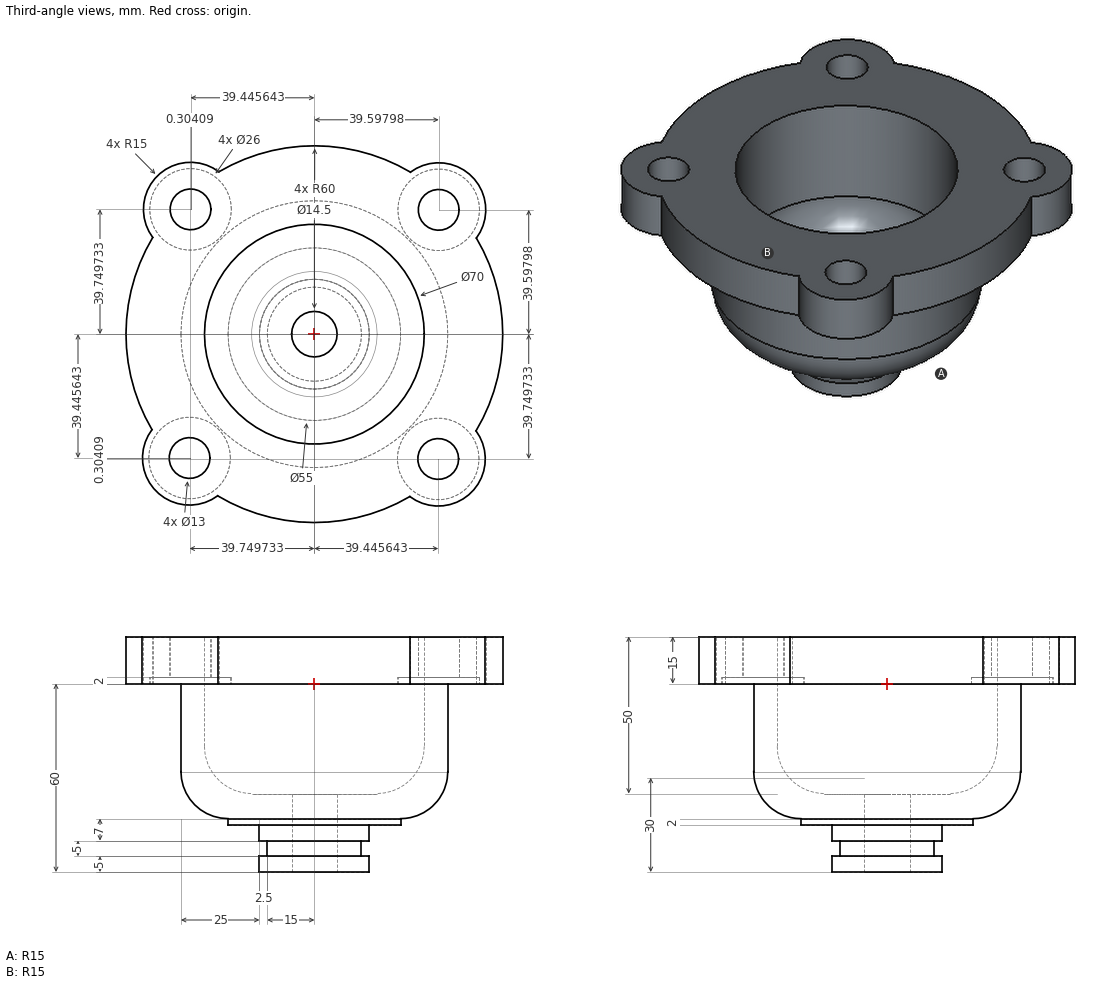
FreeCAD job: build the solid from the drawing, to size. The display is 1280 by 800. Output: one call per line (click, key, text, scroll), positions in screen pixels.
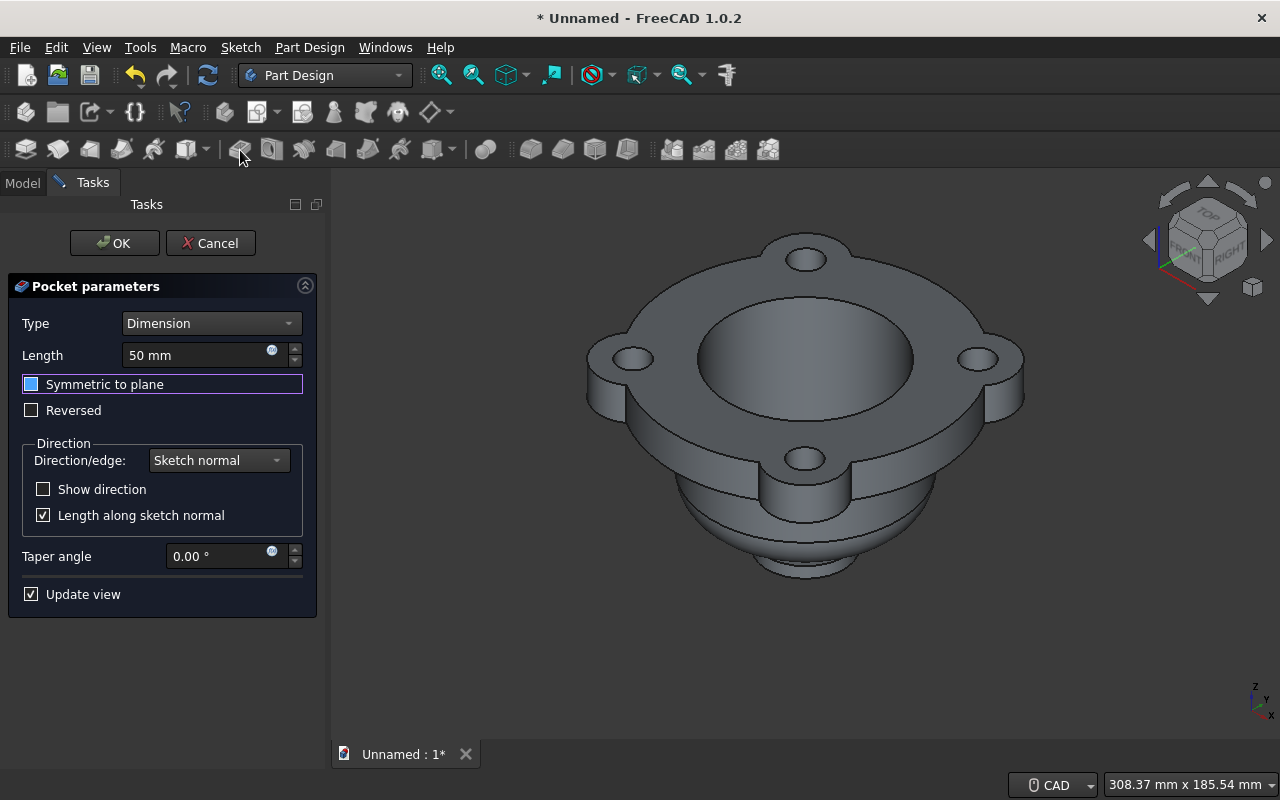
click(115, 243)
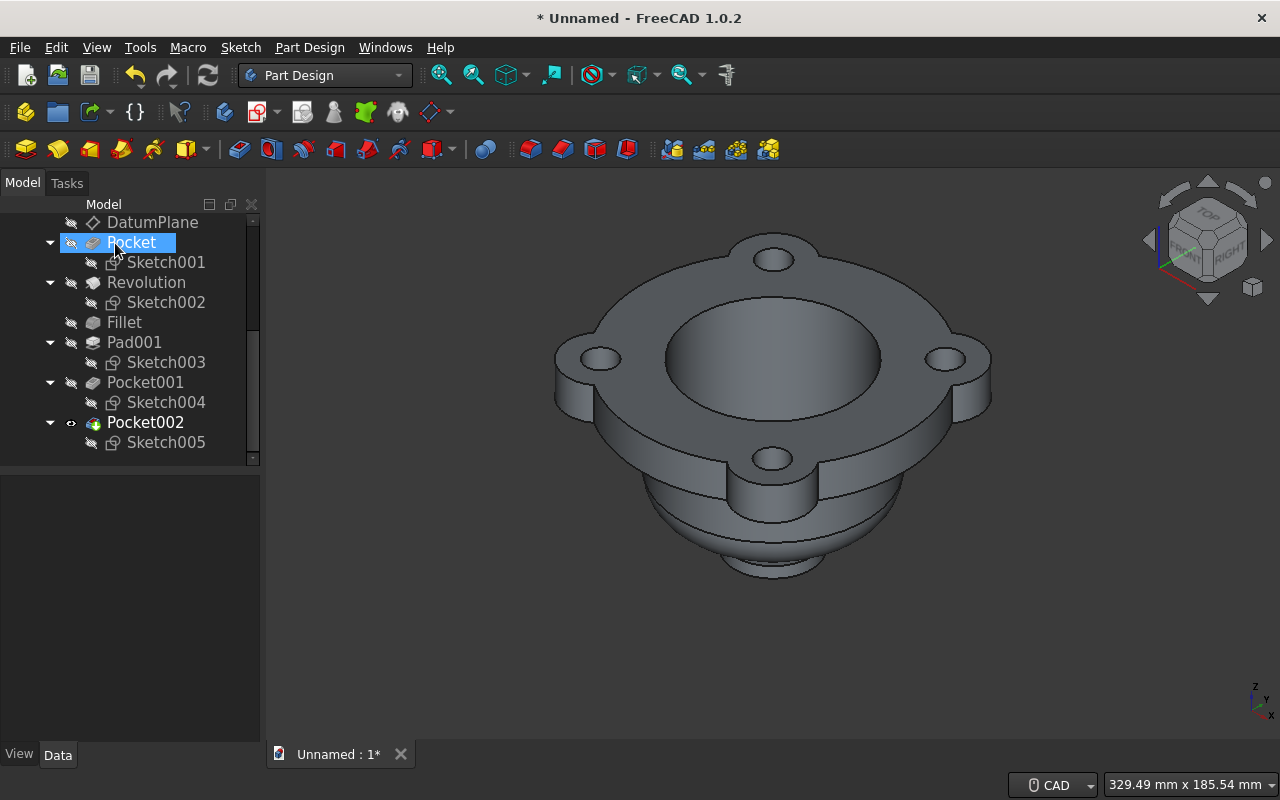
key(2)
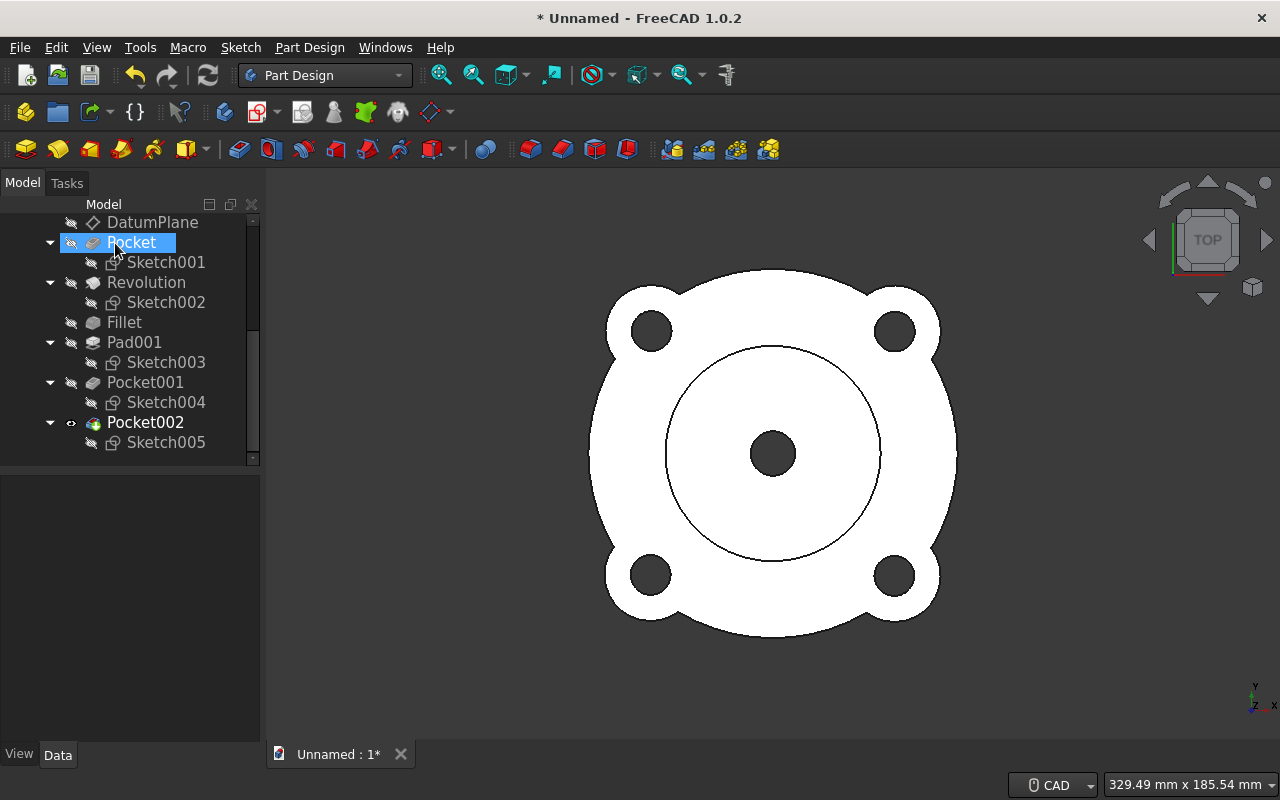
key(0)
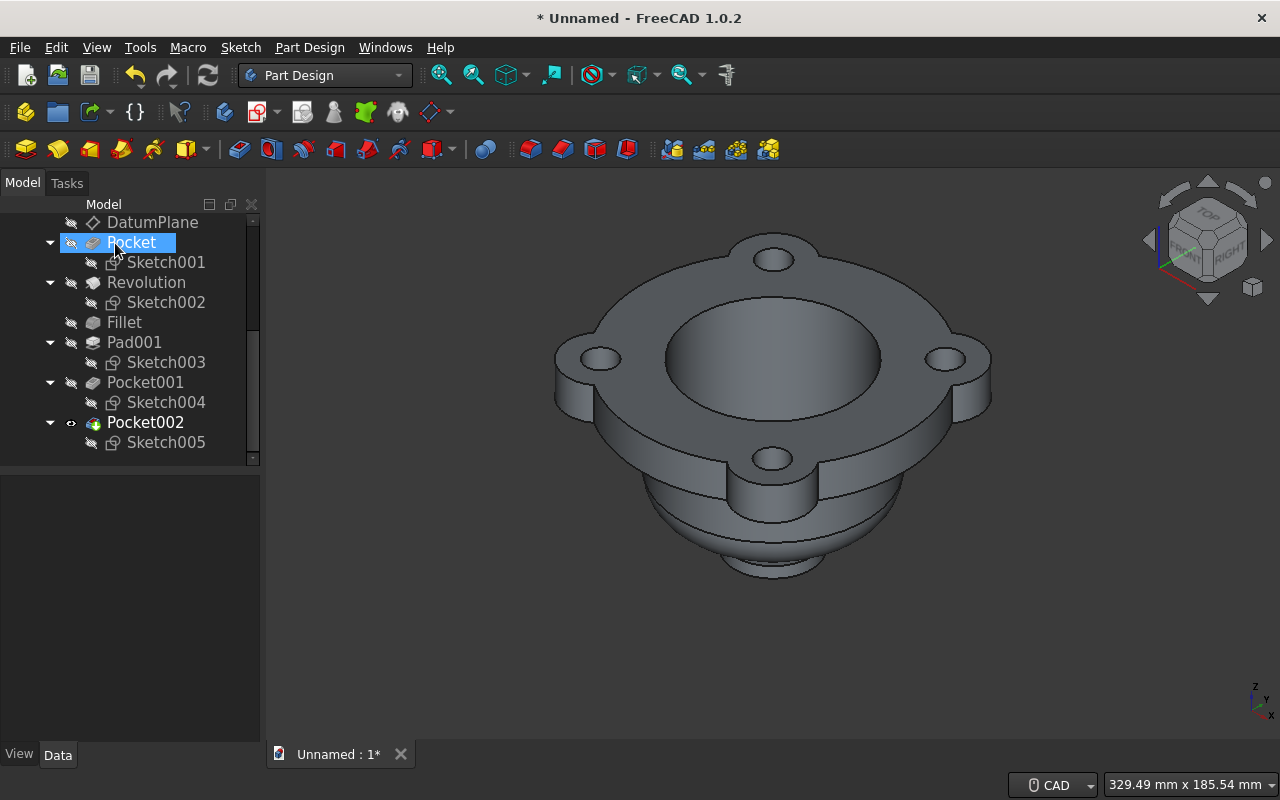
key(1)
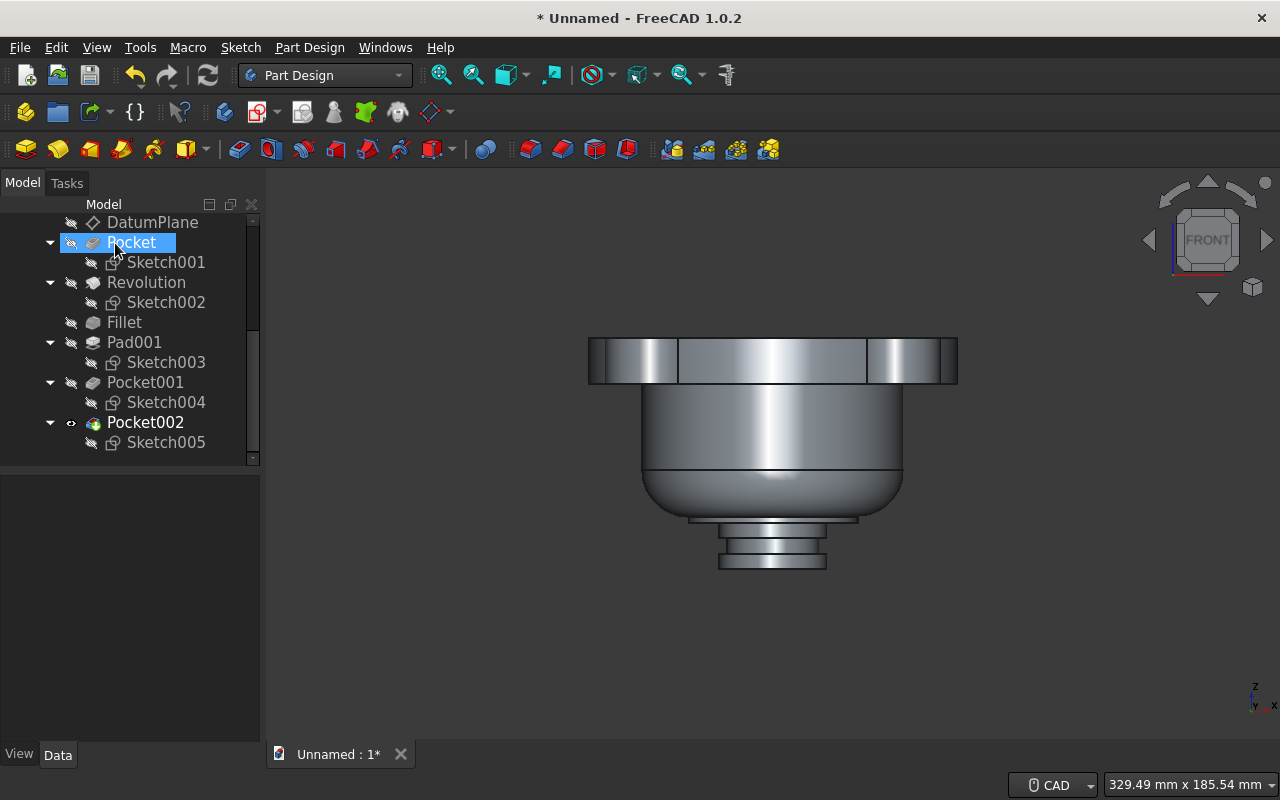
key(v)
key(f)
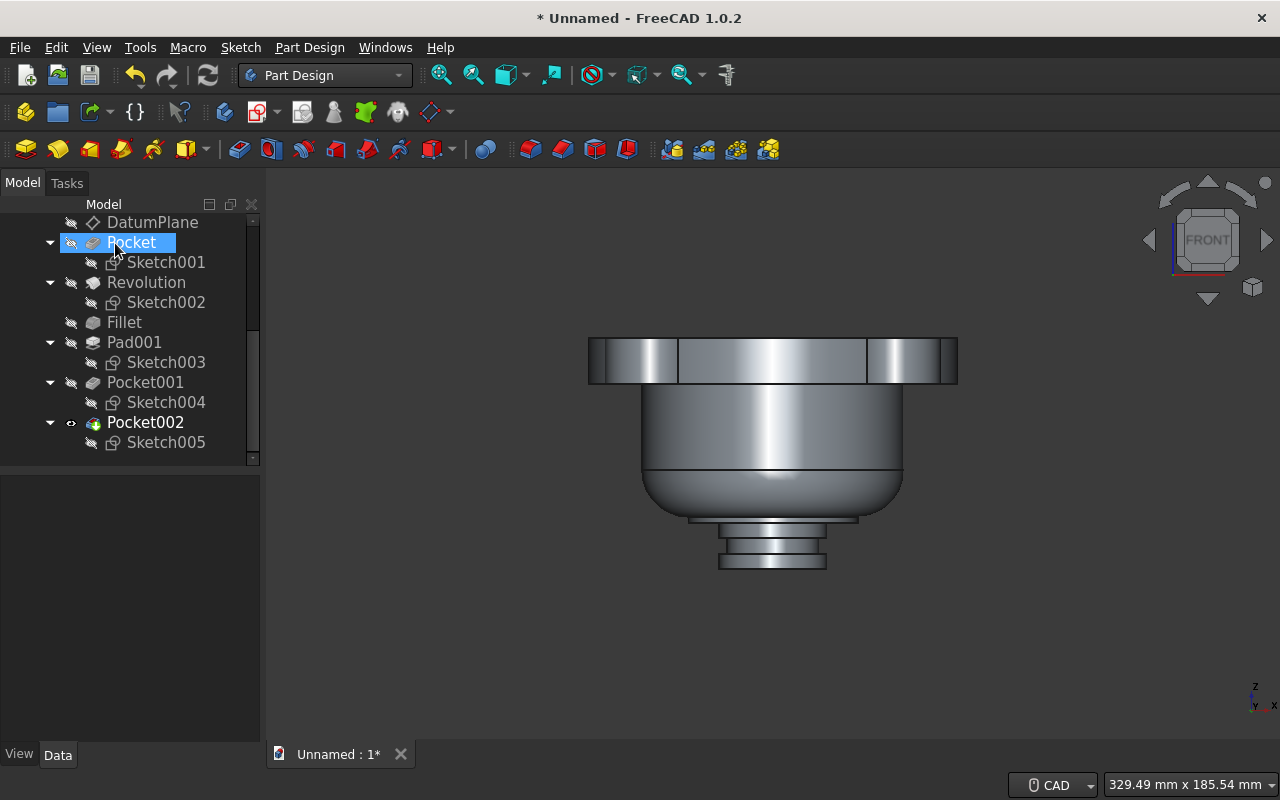
key(3)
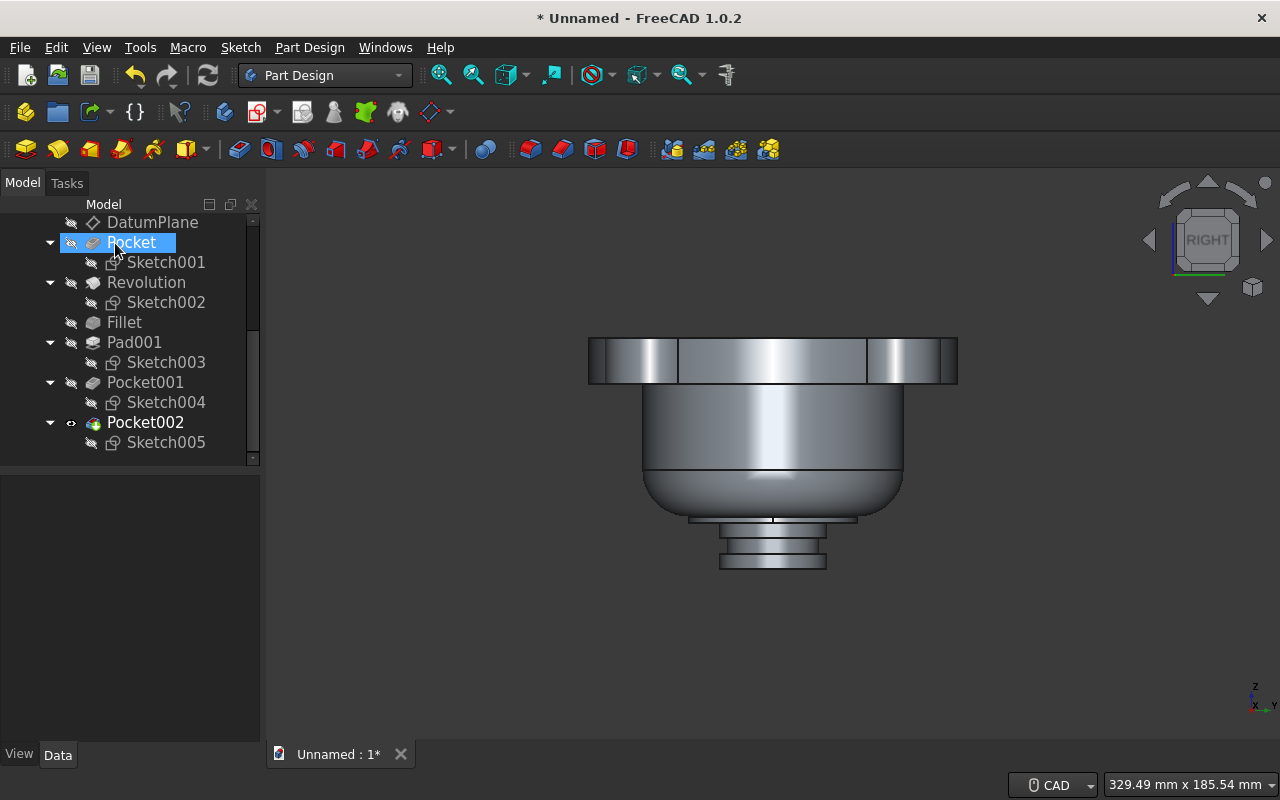
click(442, 76)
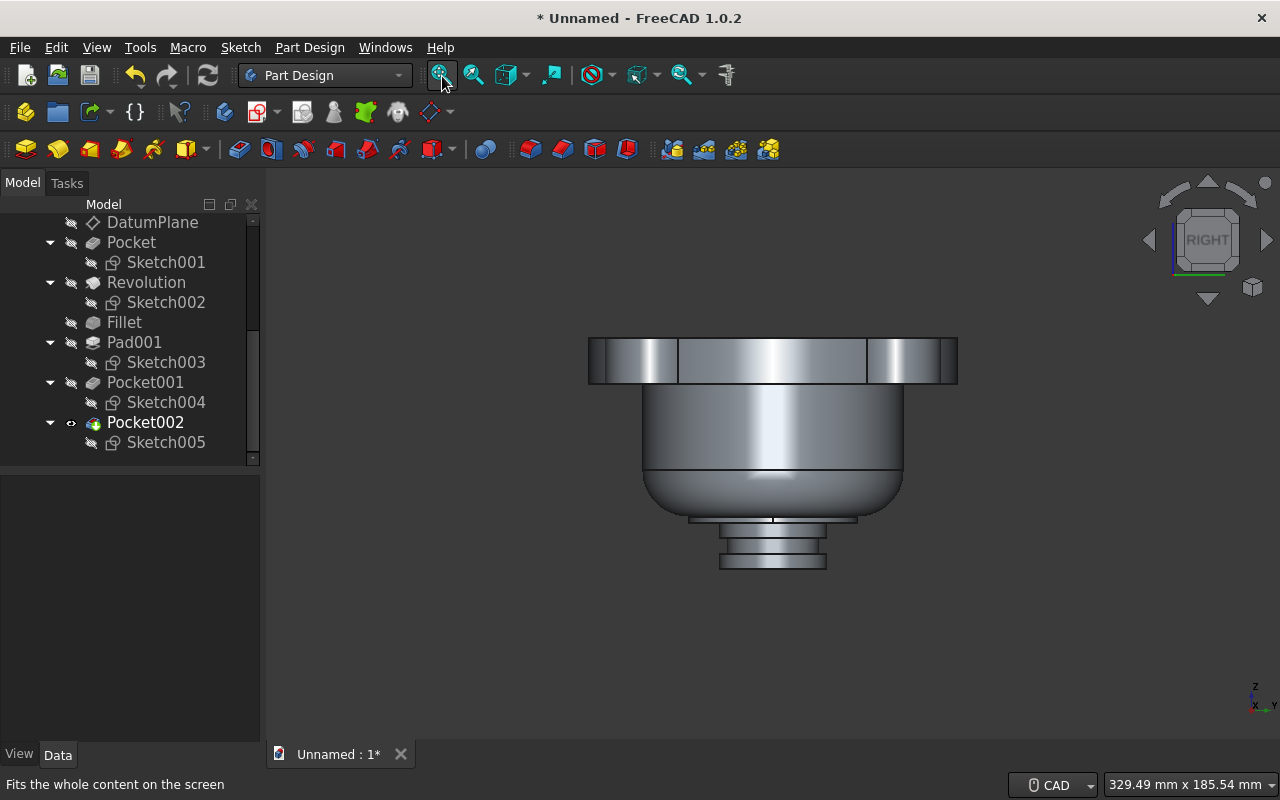
key(5)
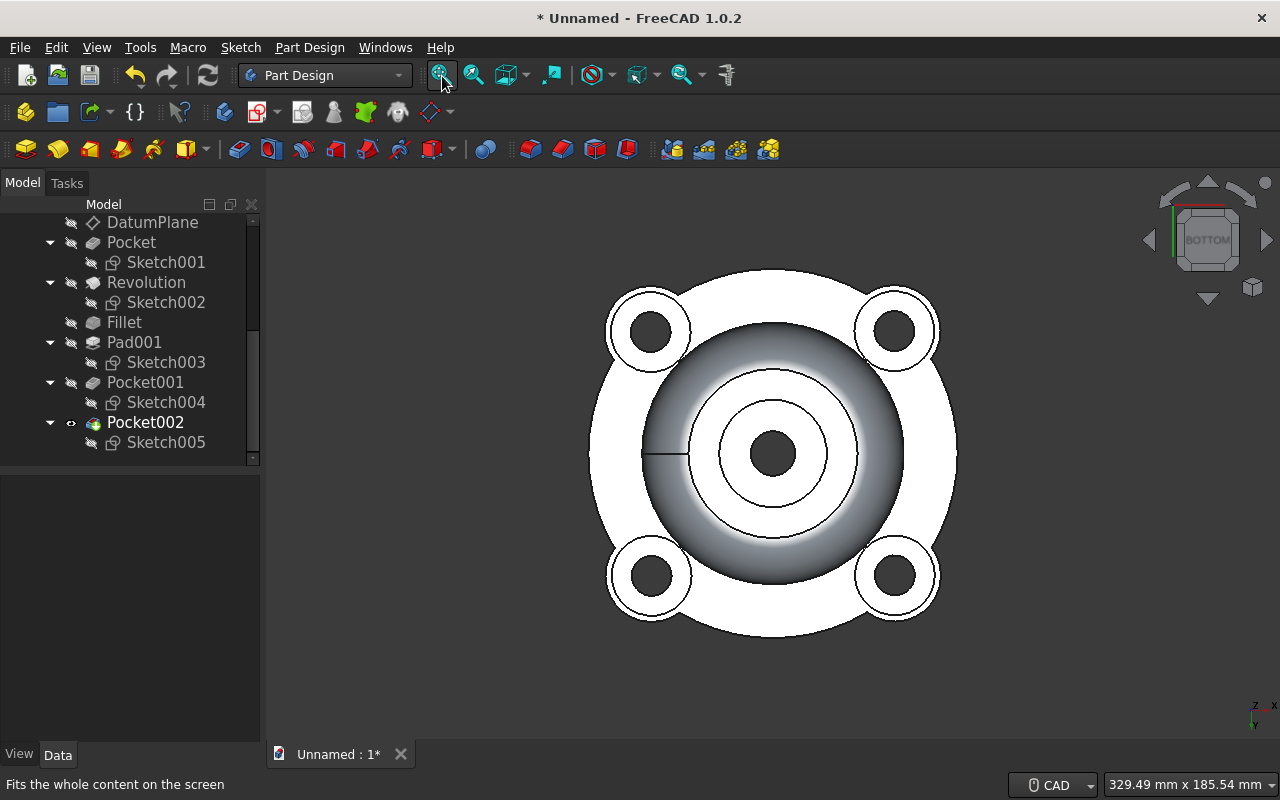
key(4)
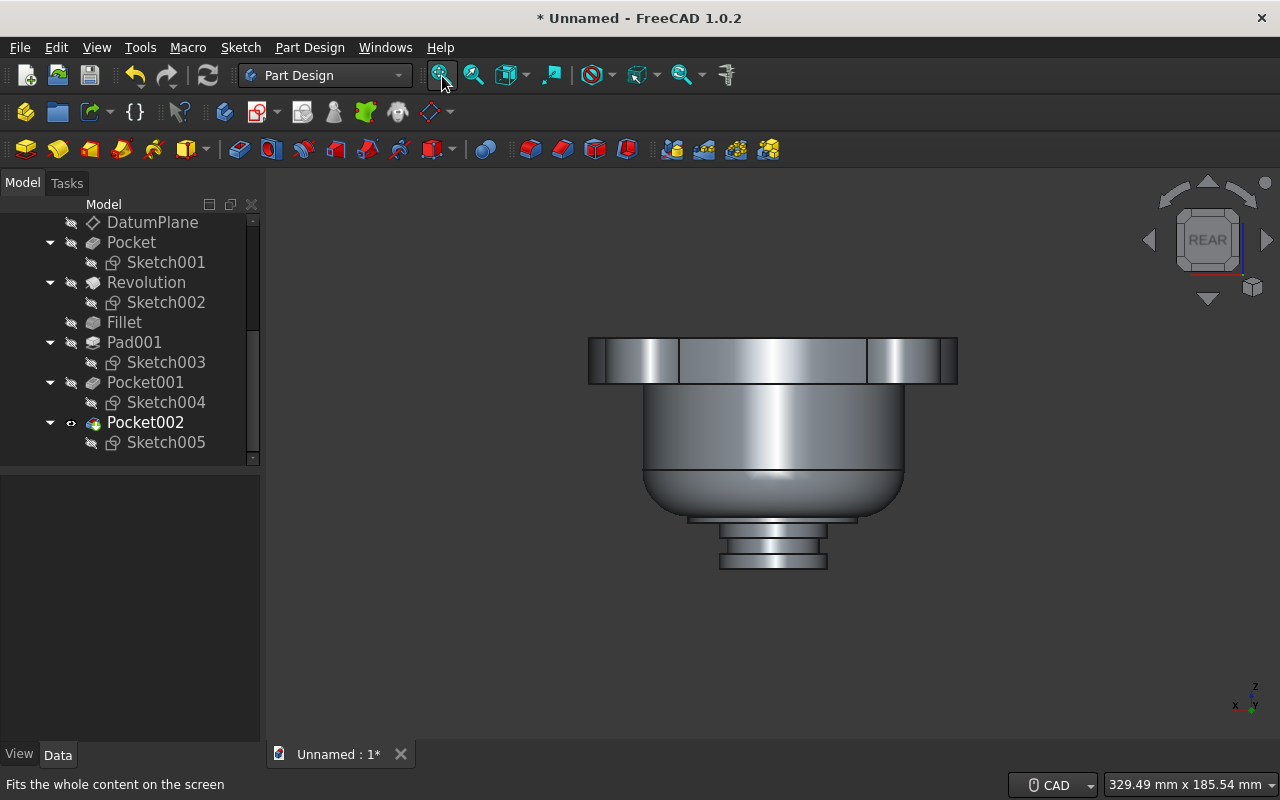
click(442, 76)